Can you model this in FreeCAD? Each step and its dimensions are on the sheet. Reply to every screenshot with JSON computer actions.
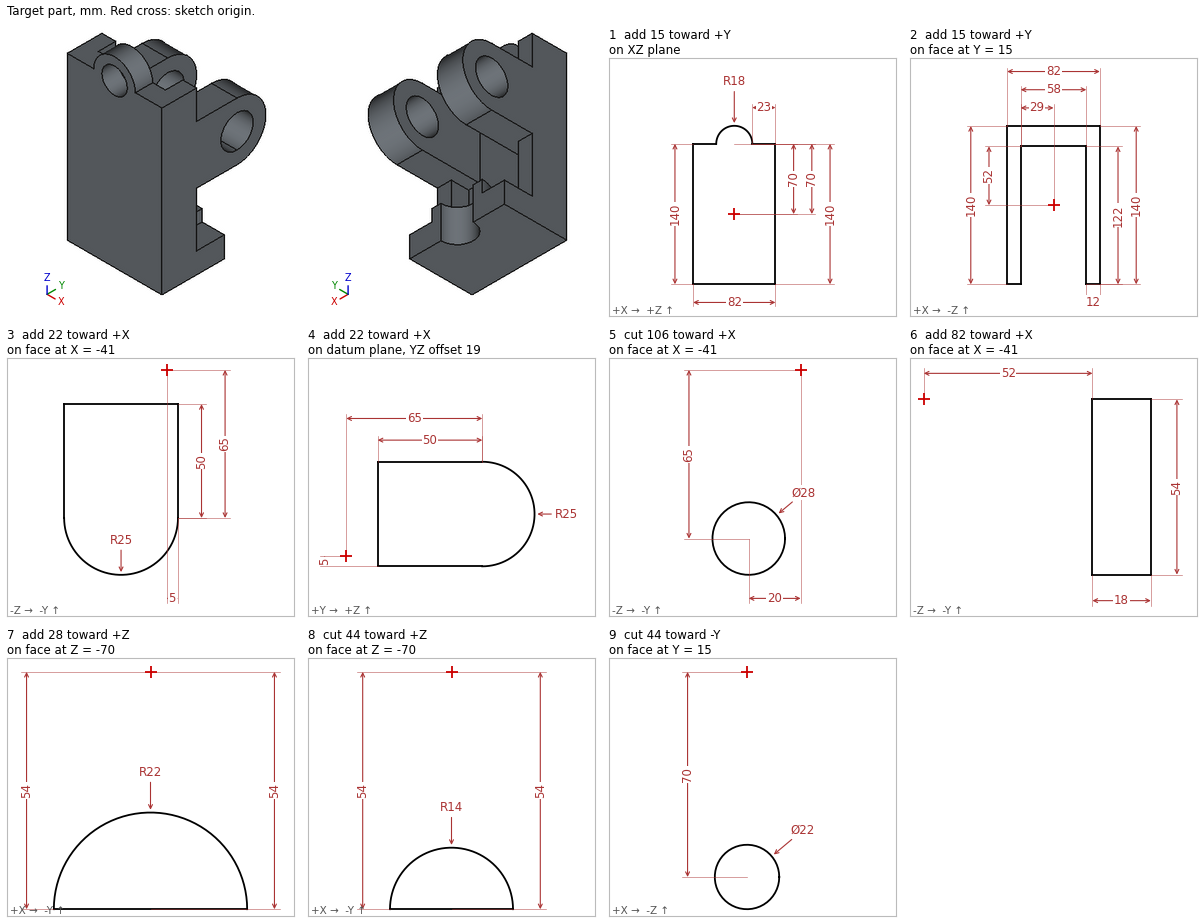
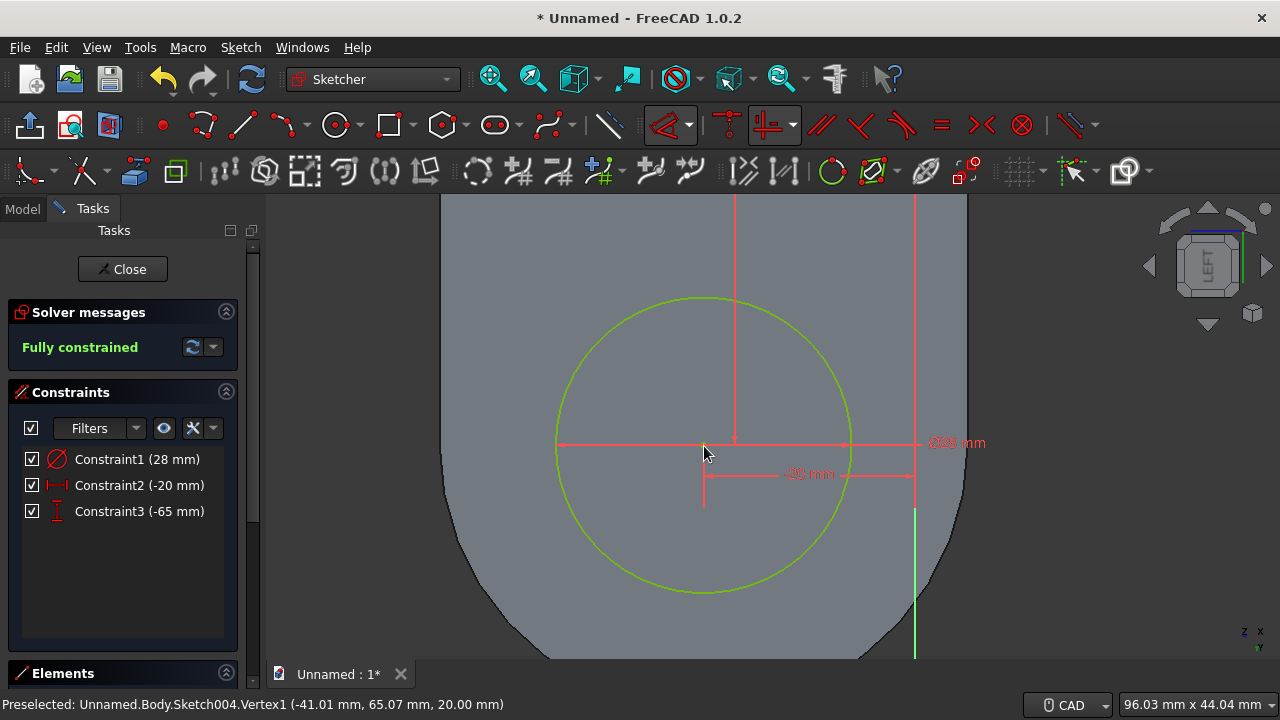
{"action": "left_click", "coordinate": [123, 269]}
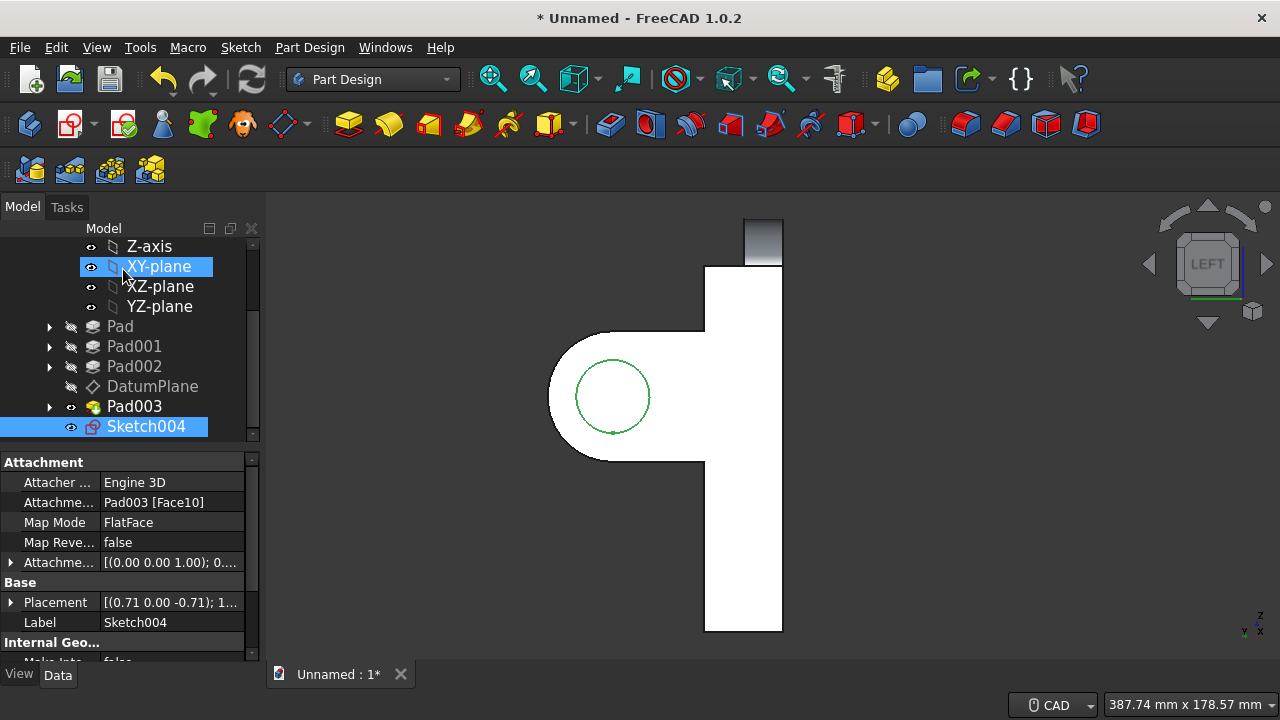
{"action": "left_click", "coordinate": [612, 124]}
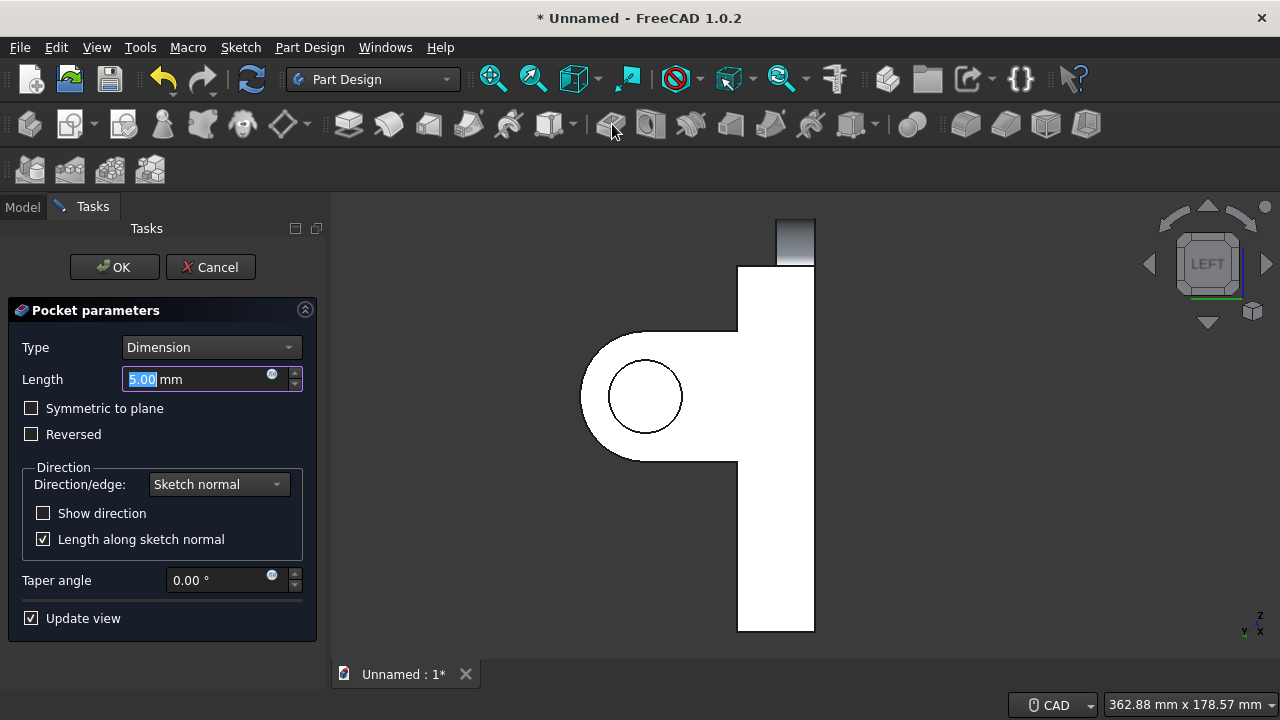
{"action": "type", "text": "106"}
{"action": "key", "text": "Tab"}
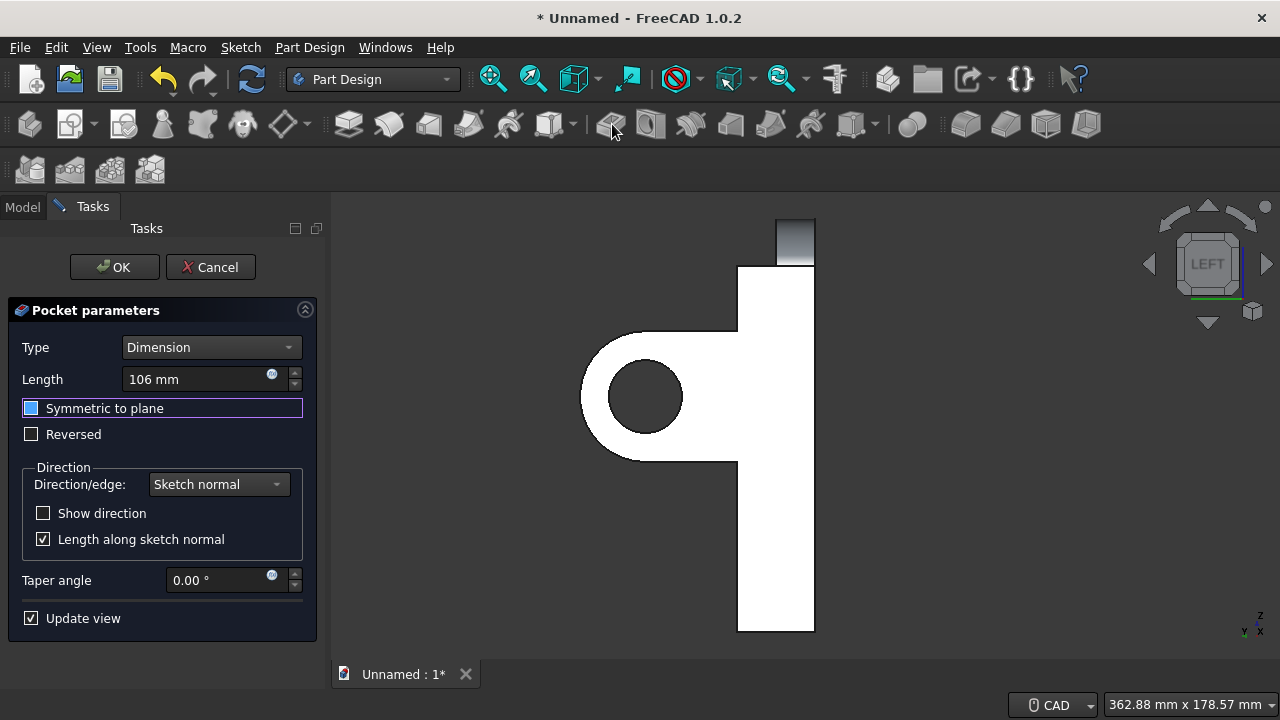
{"action": "left_click", "coordinate": [115, 267]}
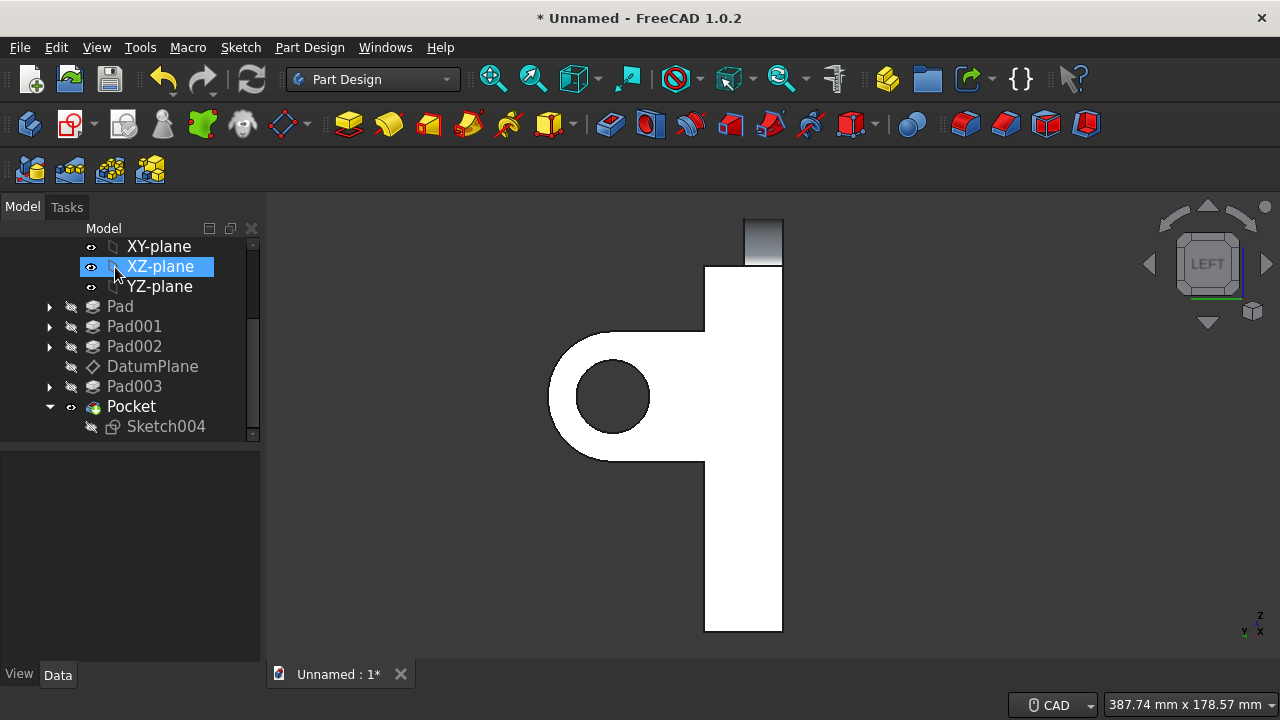
{"action": "left_click", "coordinate": [732, 396]}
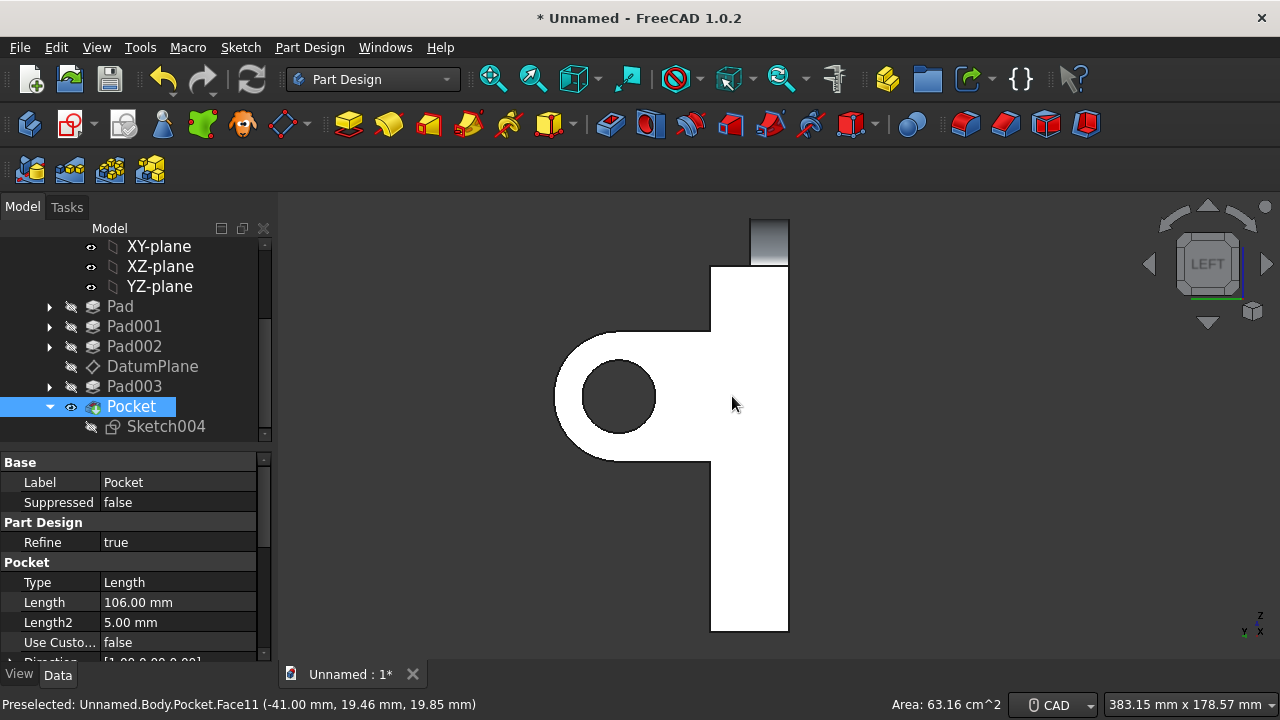
{"action": "left_click", "coordinate": [70, 124]}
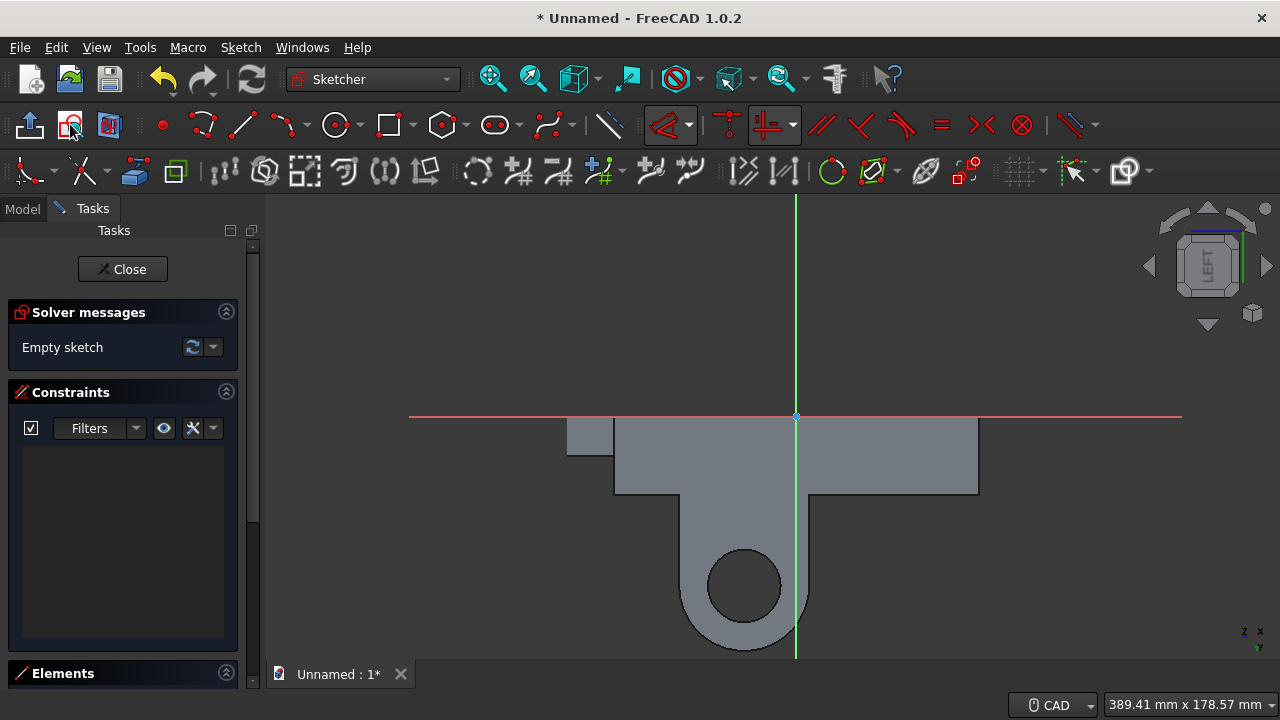
{"action": "scroll", "coordinate": [1037, 536], "scroll_direction": "up", "scroll_amount": 4}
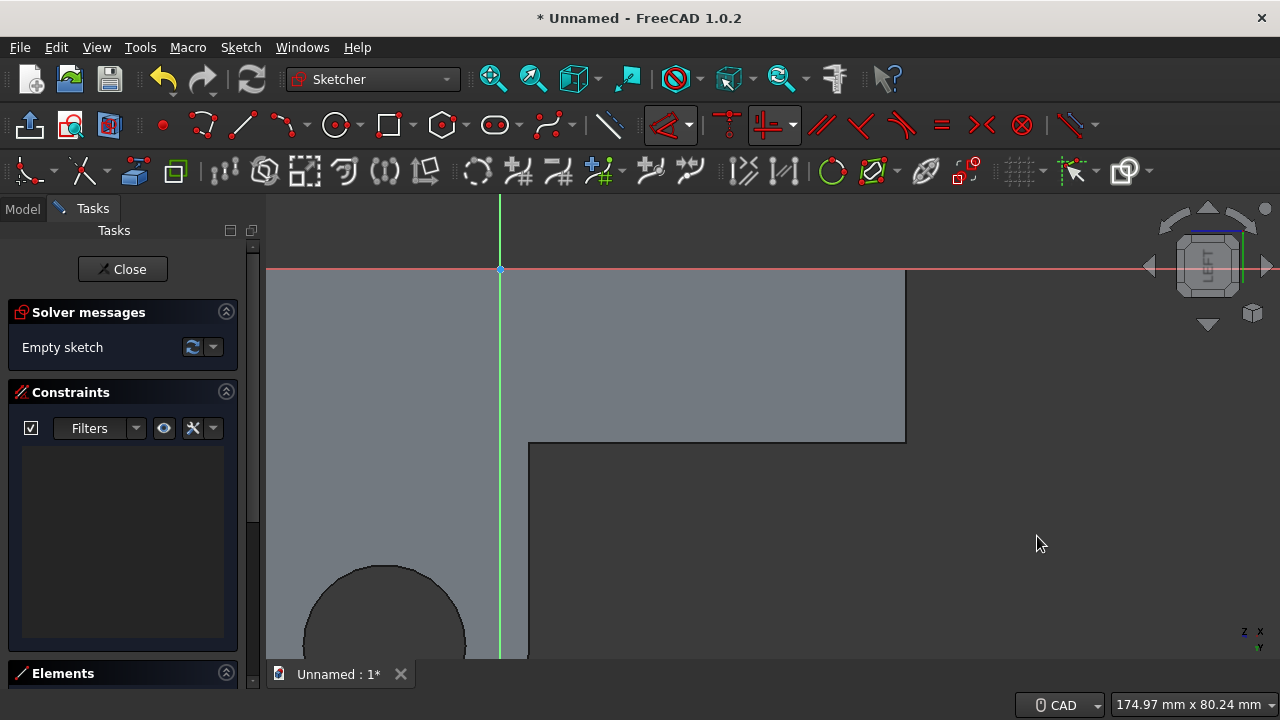
{"action": "key", "text": "g r"}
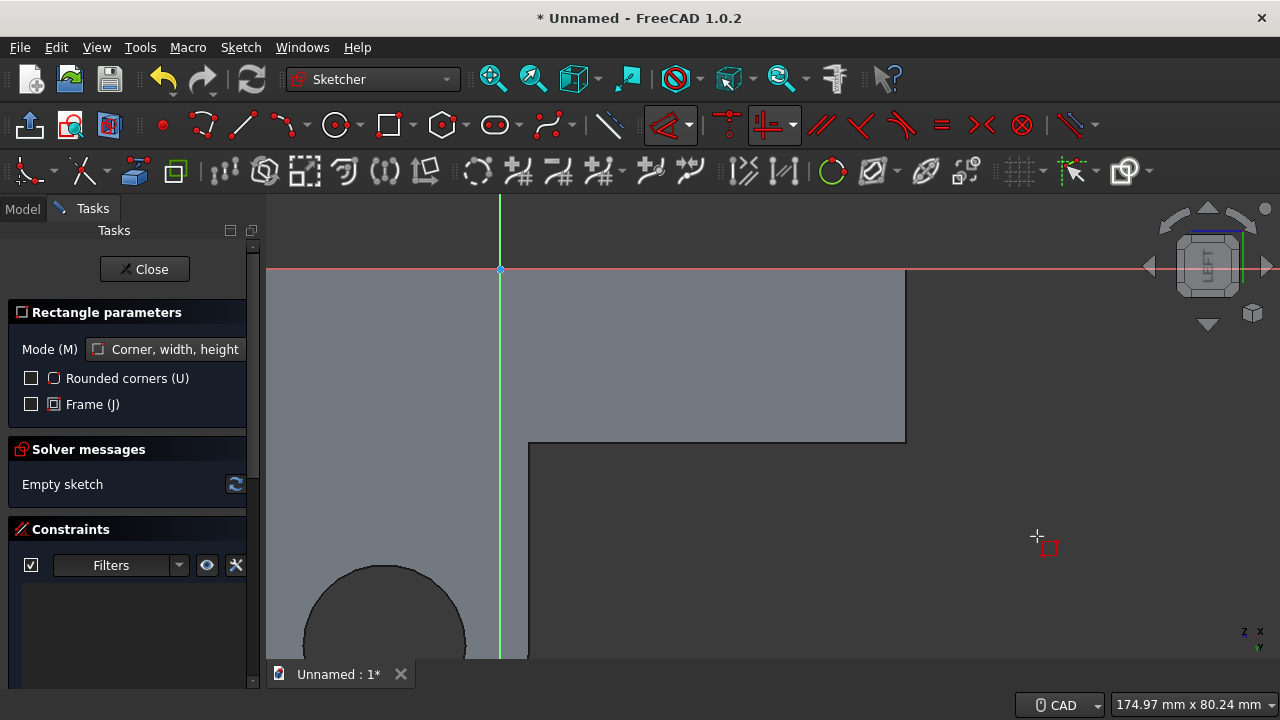
{"action": "left_click", "coordinate": [802, 269]}
{"action": "mouse_move", "coordinate": [906, 582]}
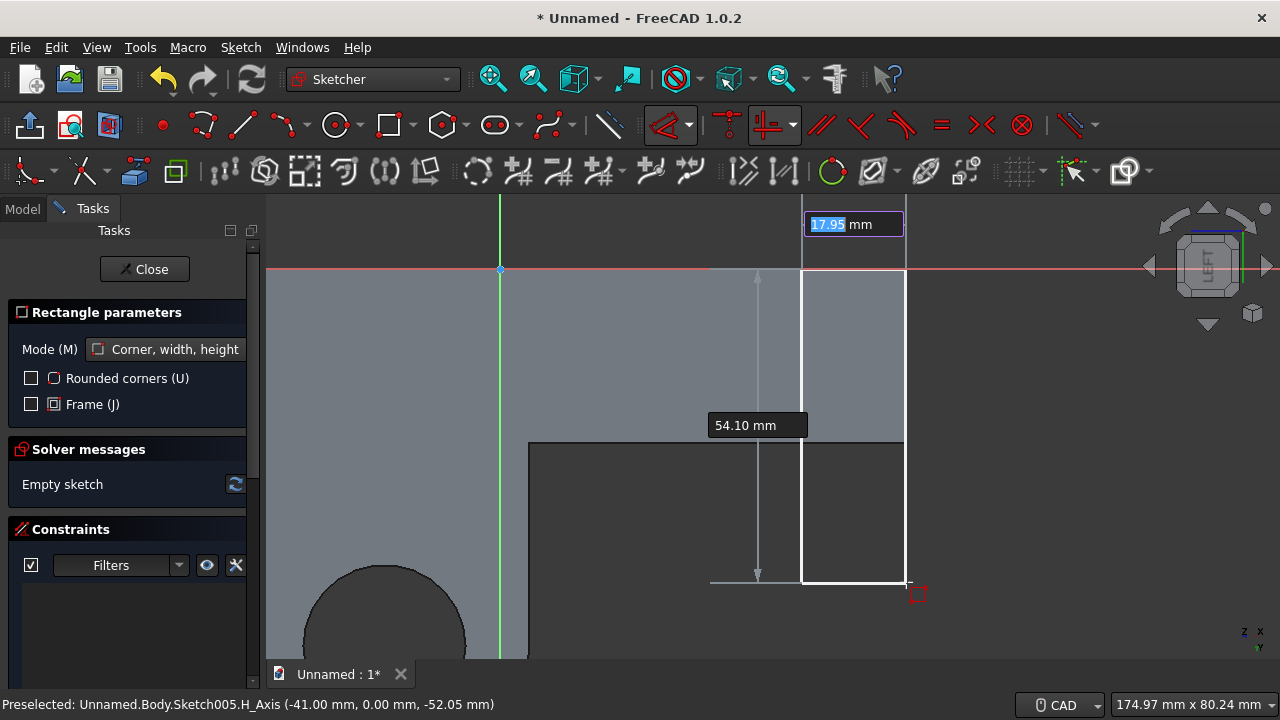
{"action": "type", "text": "18"}
{"action": "key", "text": "Tab"}
{"action": "type", "text": "54"}
{"action": "key", "text": "Return"}
{"action": "key", "text": "Escape"}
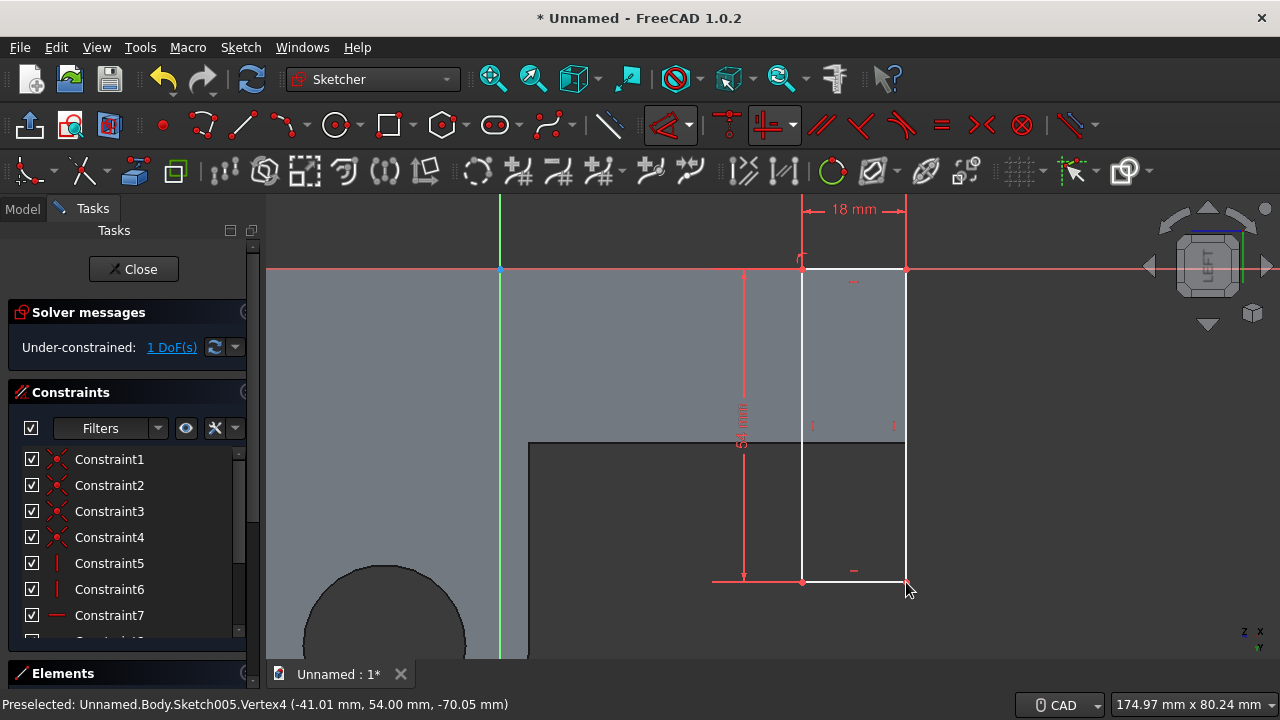
{"action": "left_click", "coordinate": [802, 269]}